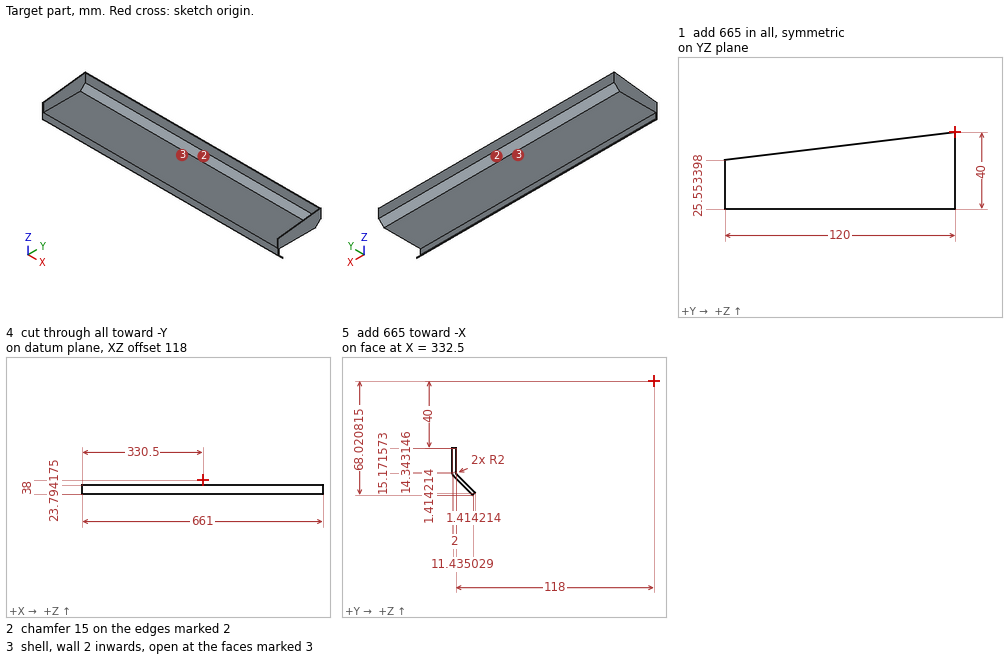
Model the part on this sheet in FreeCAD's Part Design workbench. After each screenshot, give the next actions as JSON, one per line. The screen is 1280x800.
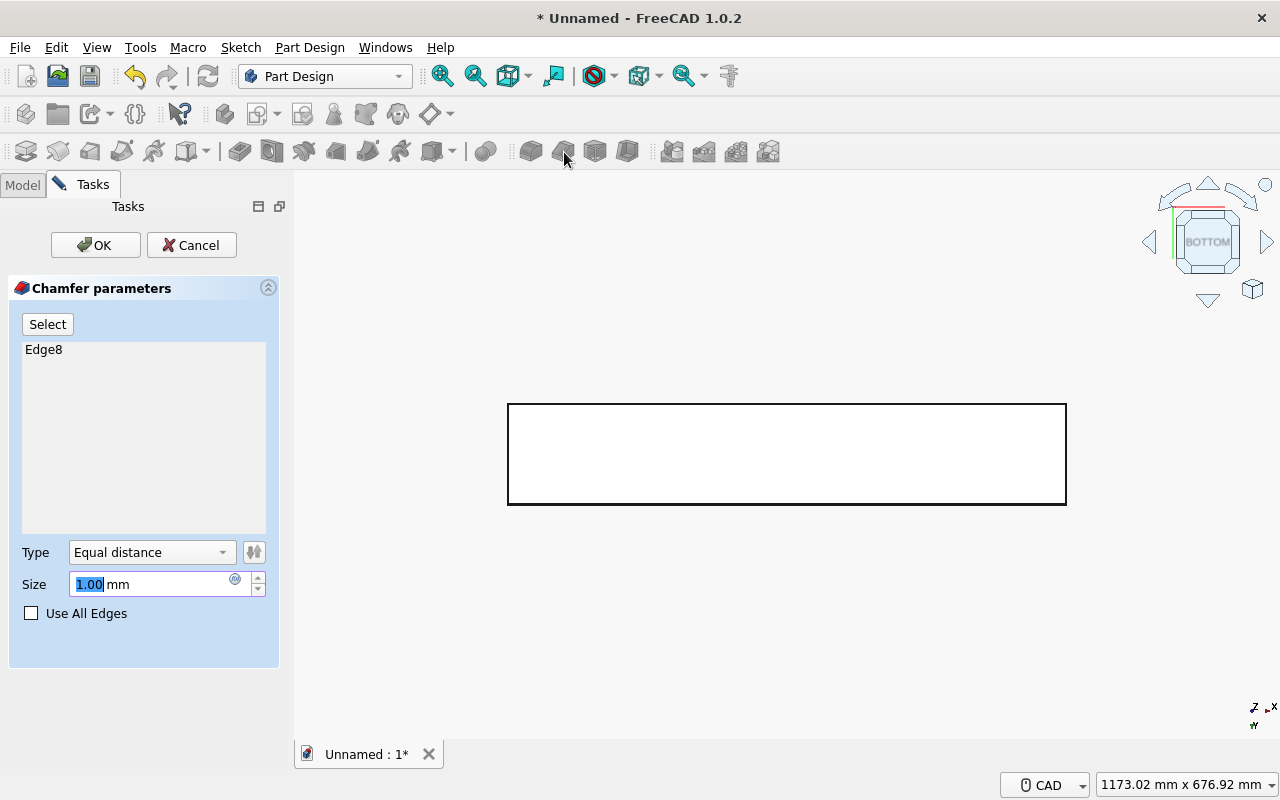
{"action": "type", "text": "15"}
{"action": "key", "text": "Tab"}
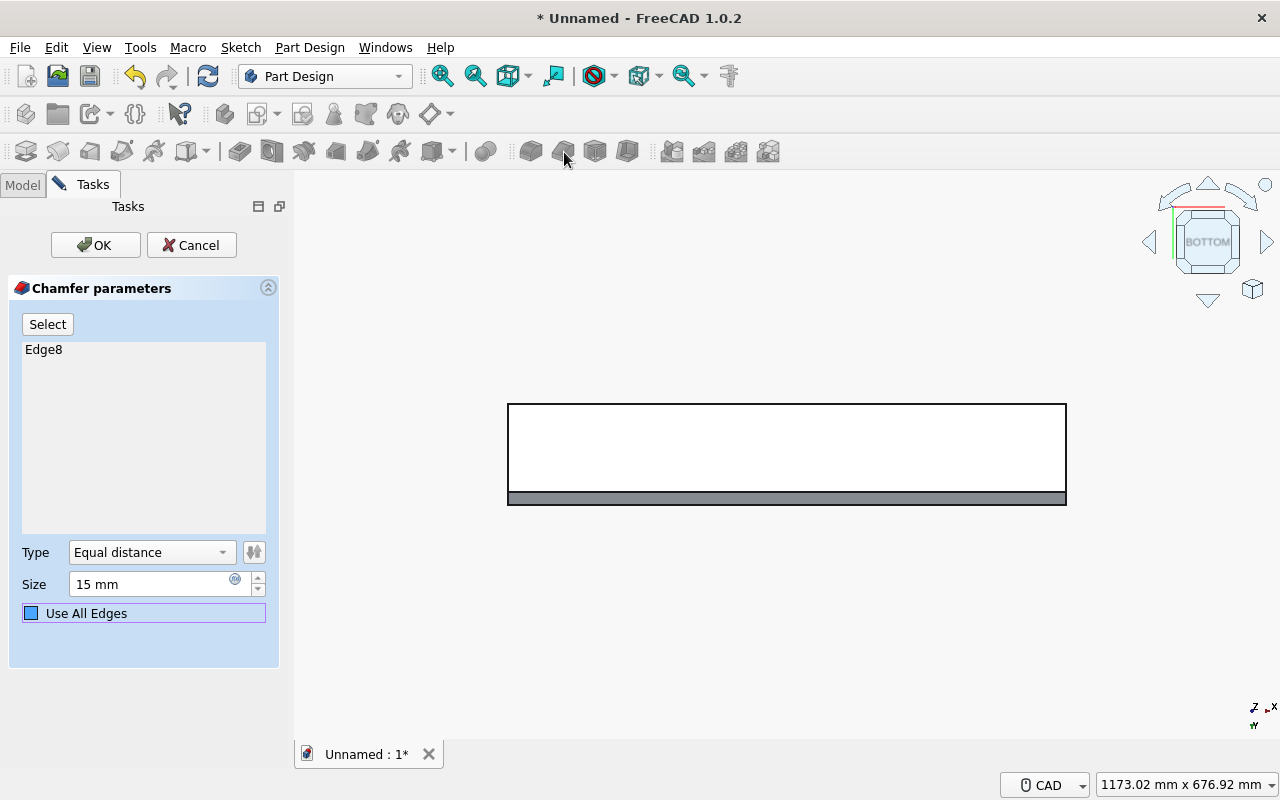
{"action": "left_click", "coordinate": [96, 245]}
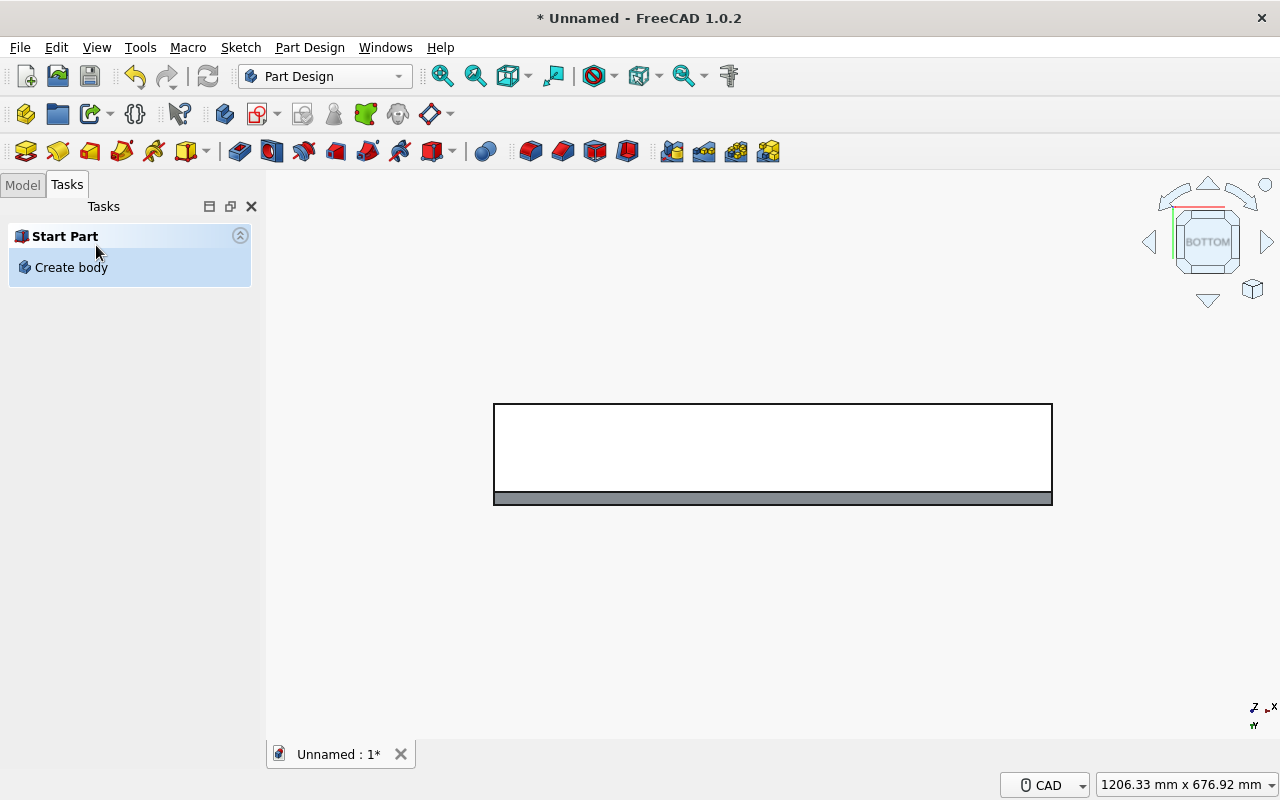
{"action": "key", "text": "0"}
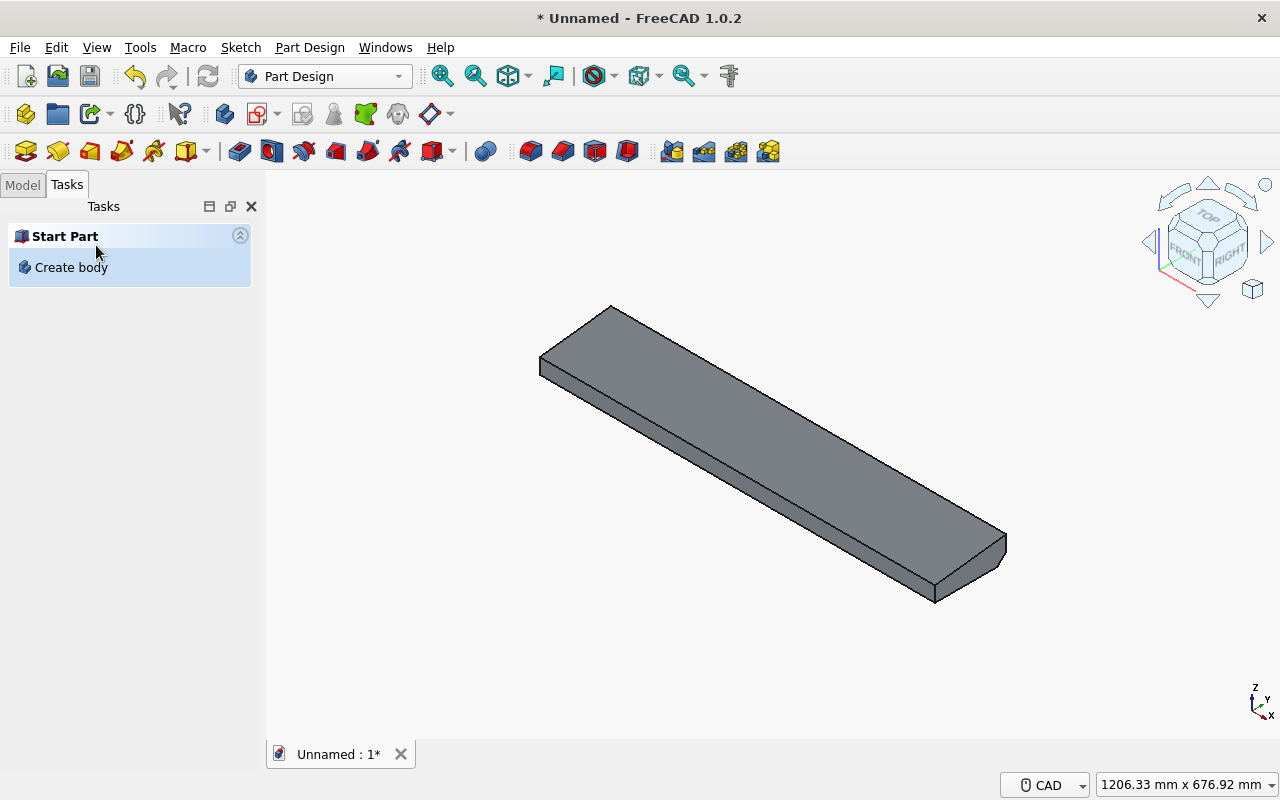
{"action": "left_click", "coordinate": [773, 445]}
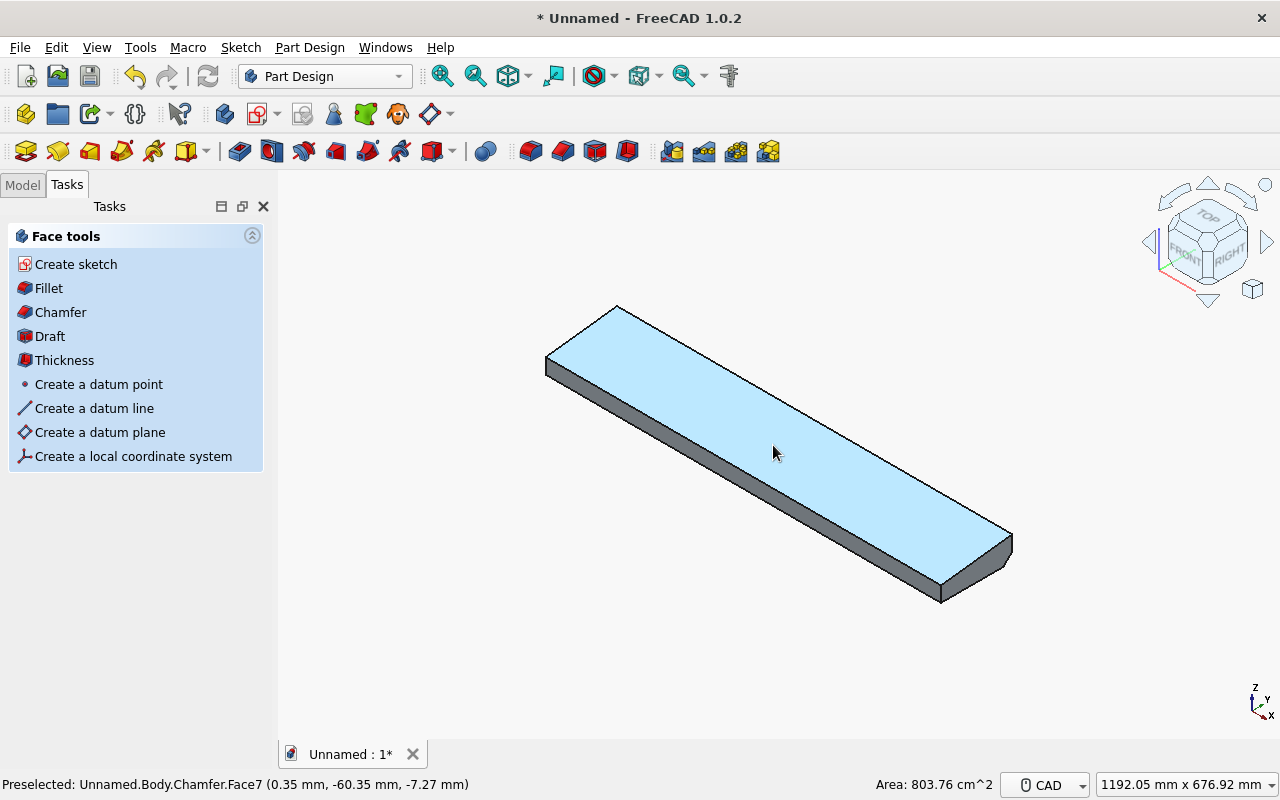
{"action": "left_click", "coordinate": [628, 152]}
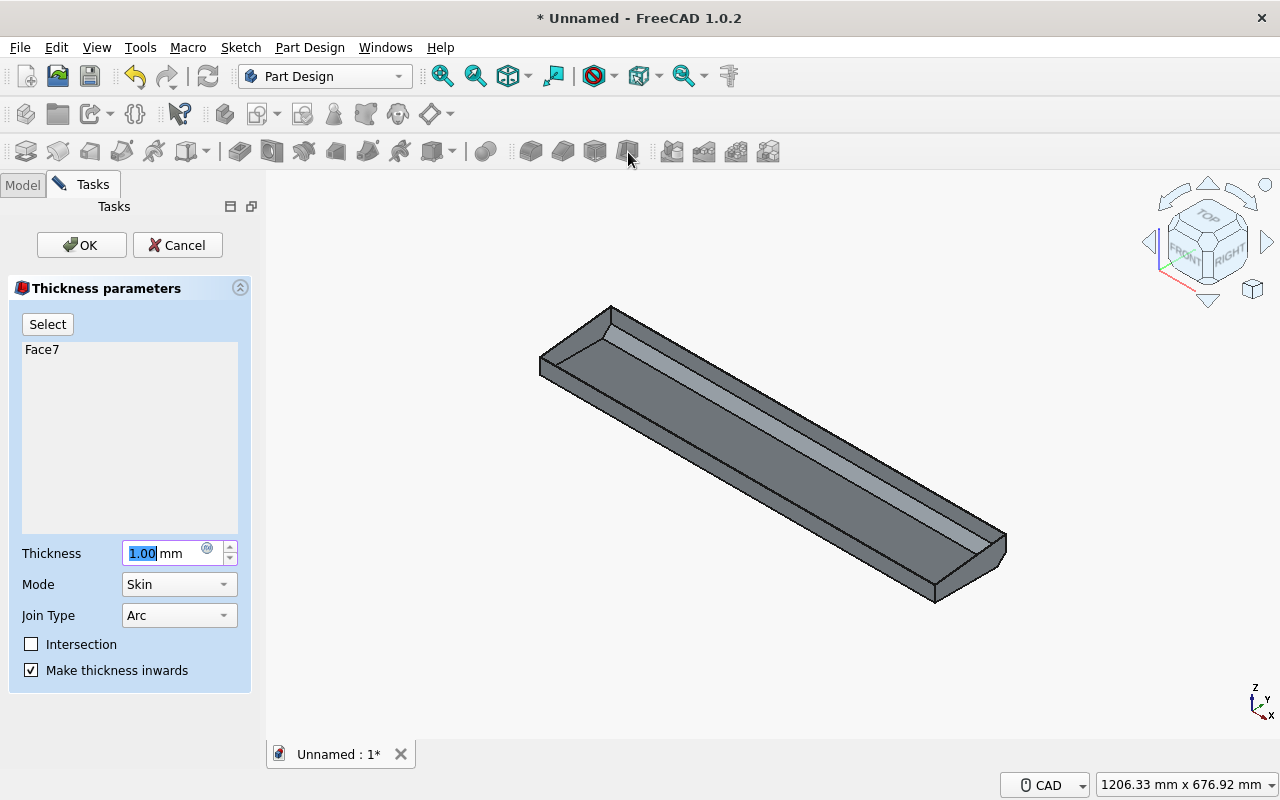
{"action": "type", "text": "2"}
{"action": "key", "text": "Tab"}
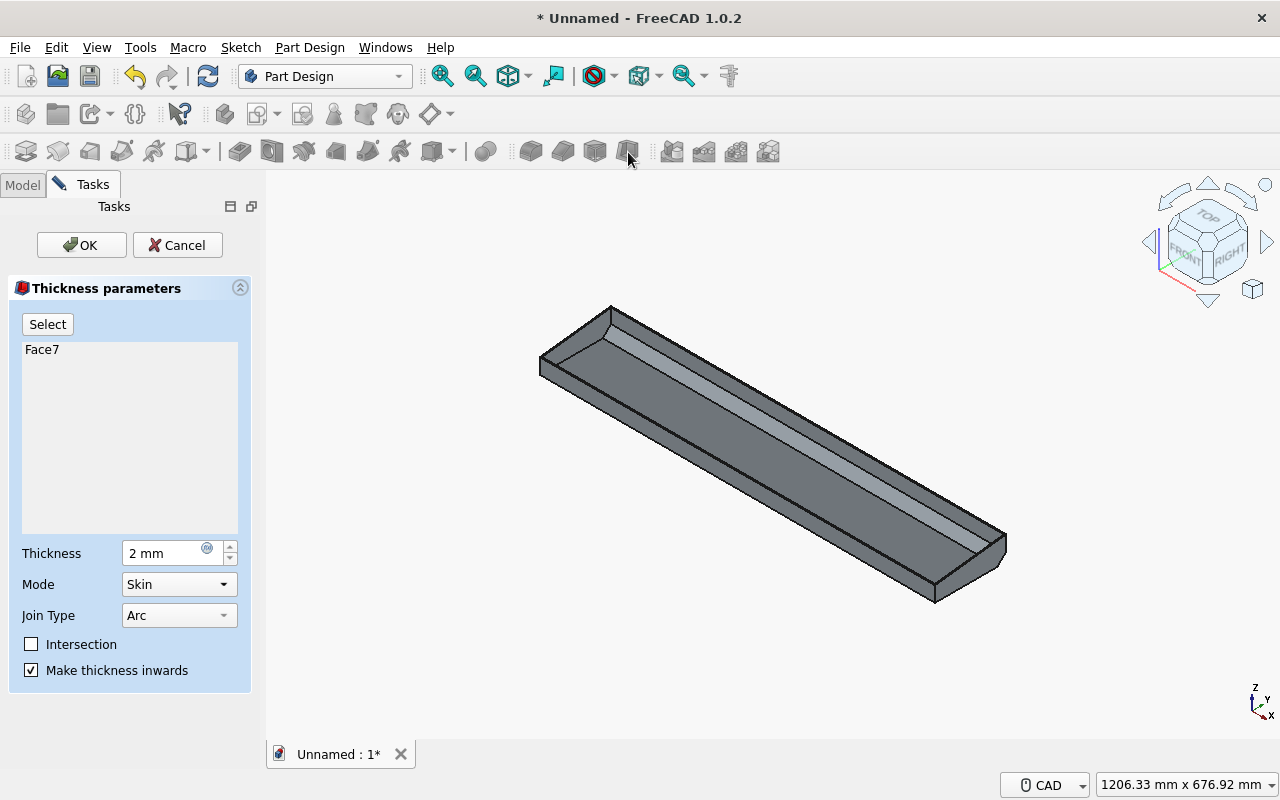
{"action": "left_click", "coordinate": [180, 616]}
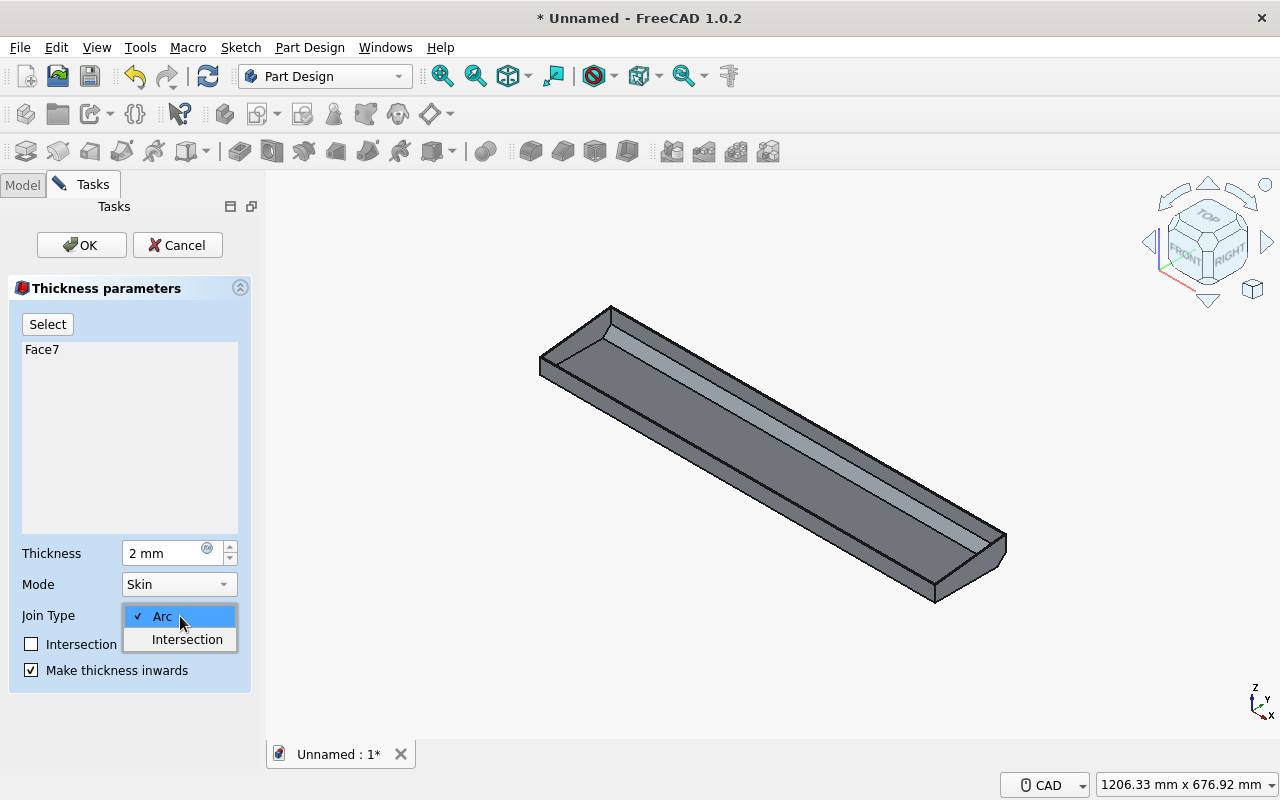
{"action": "left_click", "coordinate": [179, 640]}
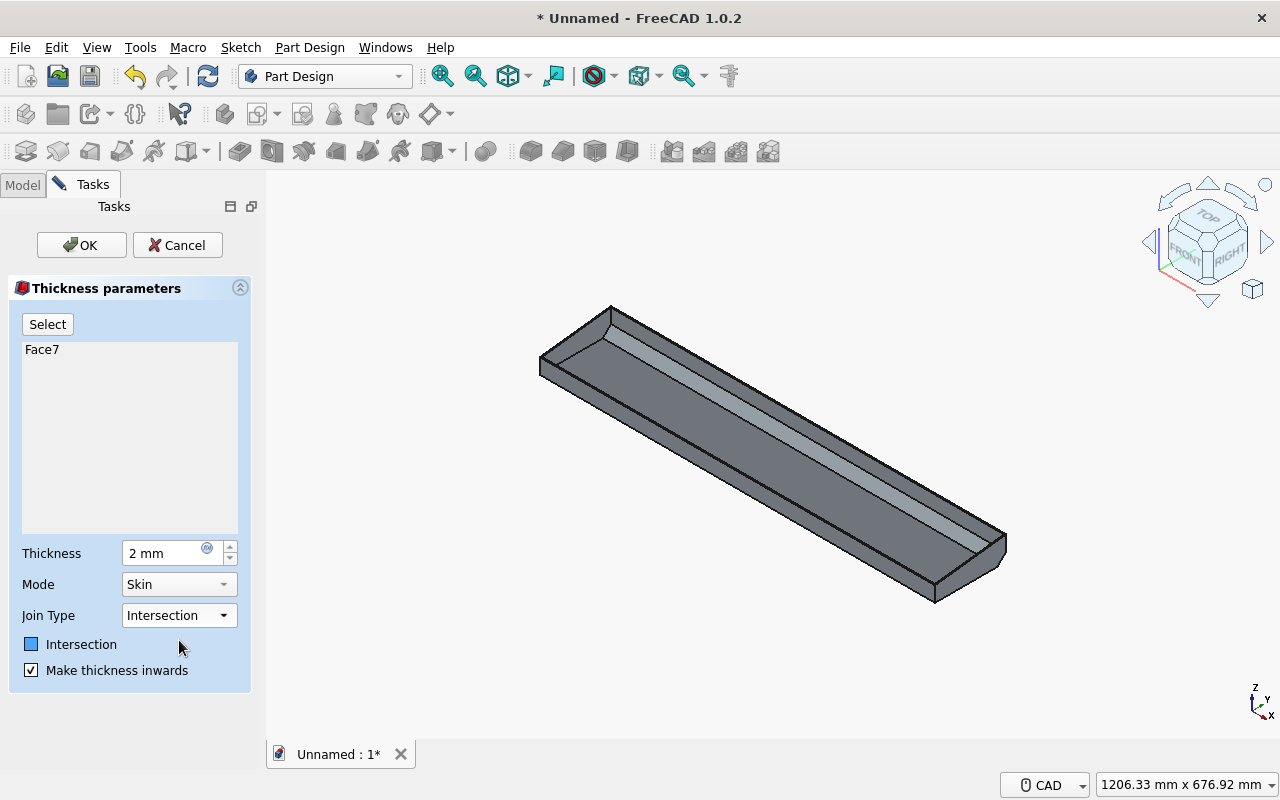
{"action": "left_click", "coordinate": [82, 245]}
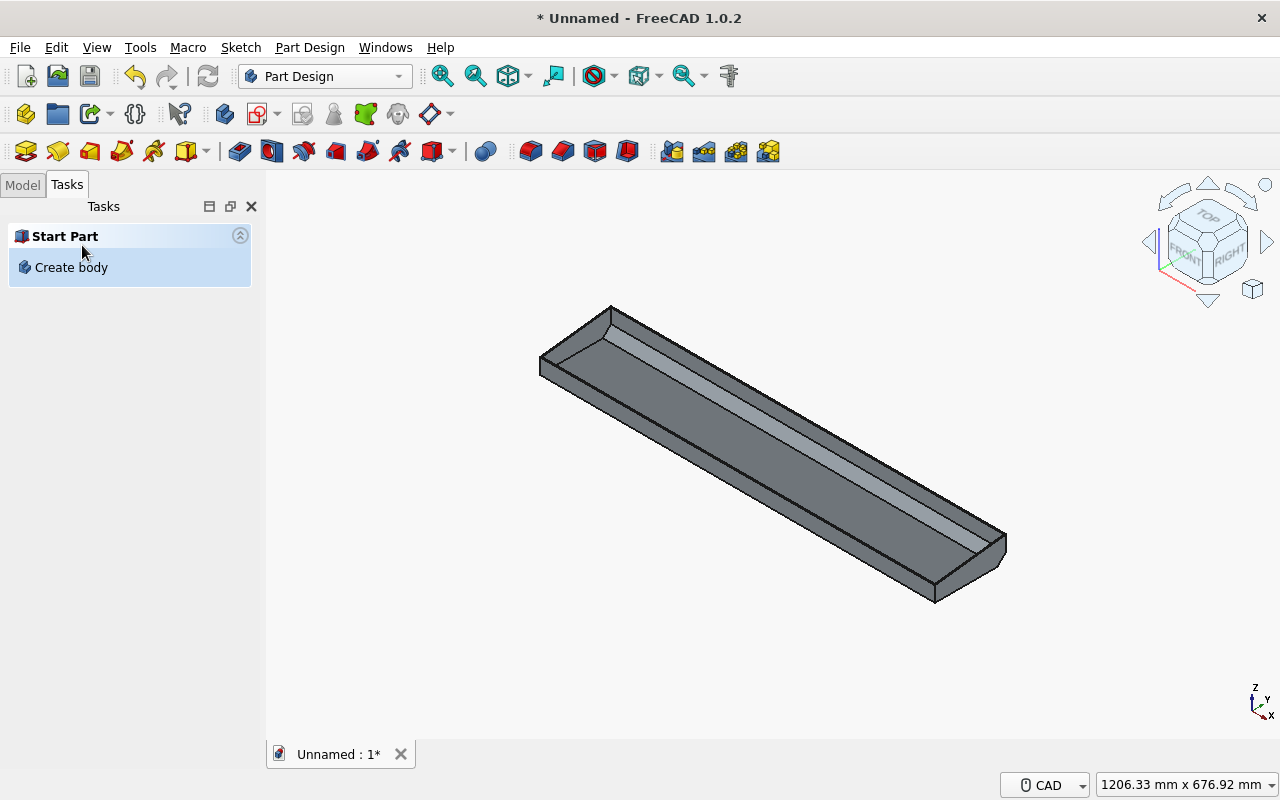
{"action": "left_click", "coordinate": [23, 184]}